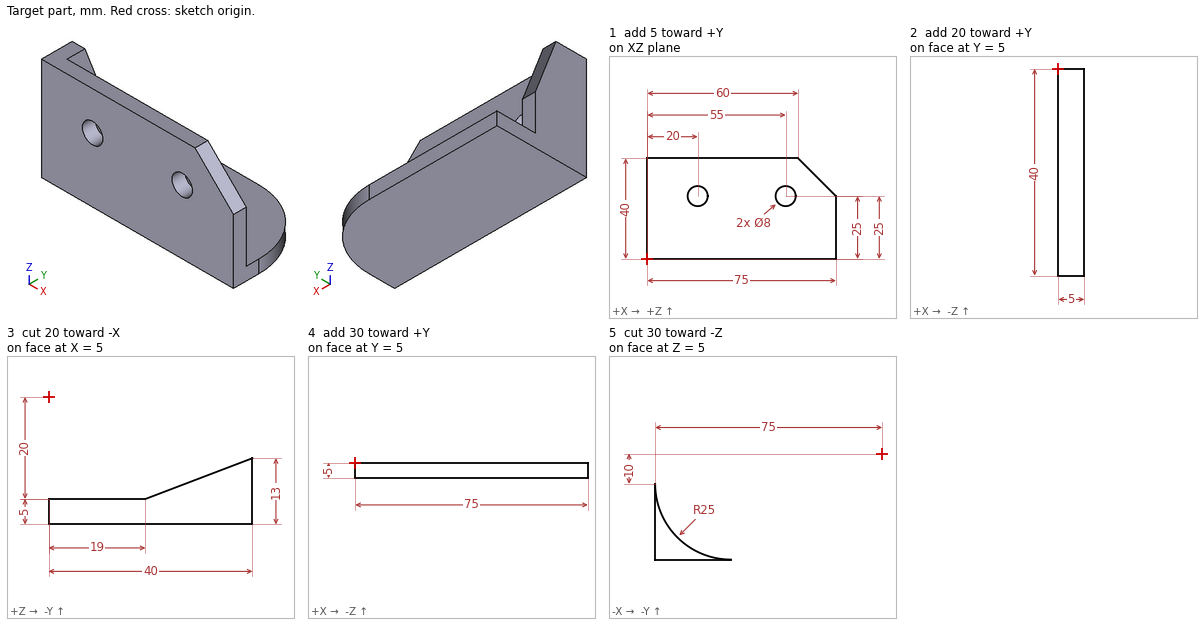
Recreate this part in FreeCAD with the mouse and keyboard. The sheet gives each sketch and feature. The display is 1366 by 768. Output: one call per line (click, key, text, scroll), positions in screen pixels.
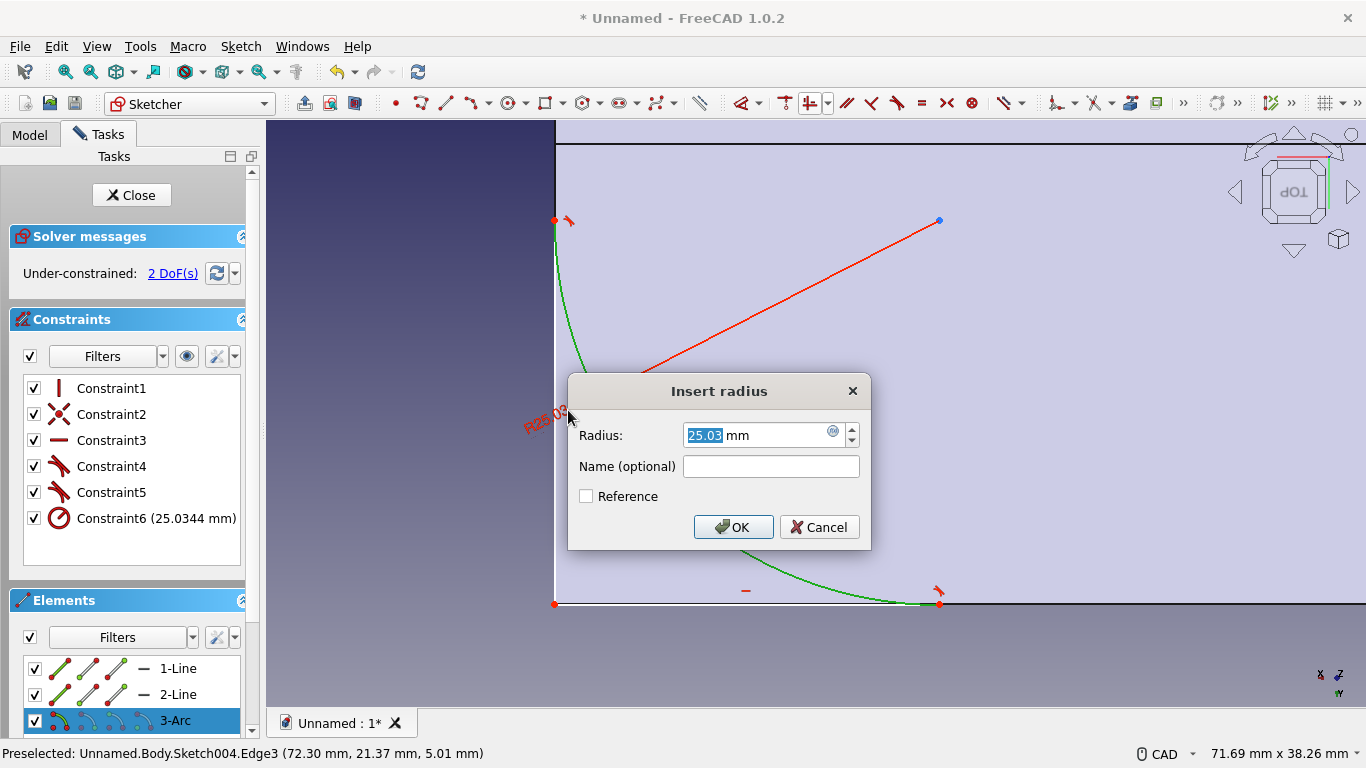
text(25)
key(Return)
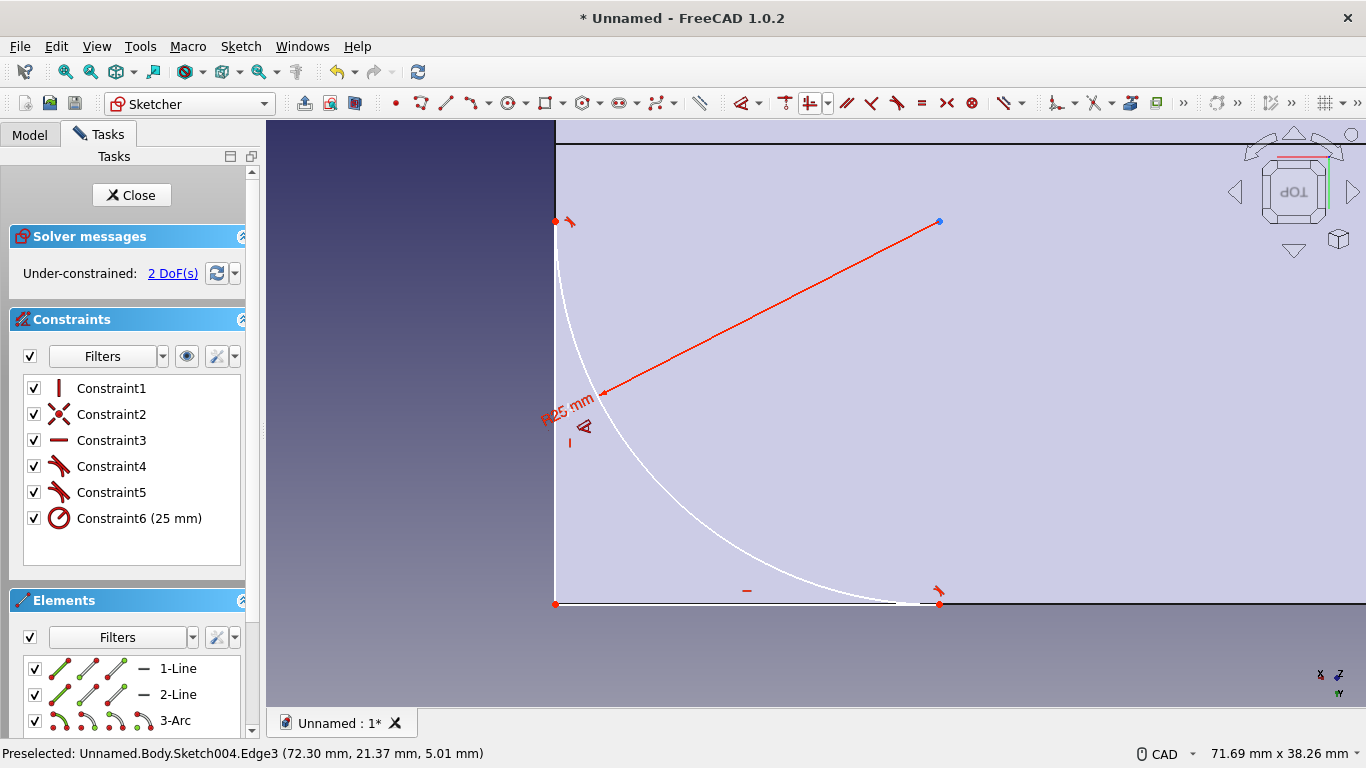
click(555, 221)
click(878, 255)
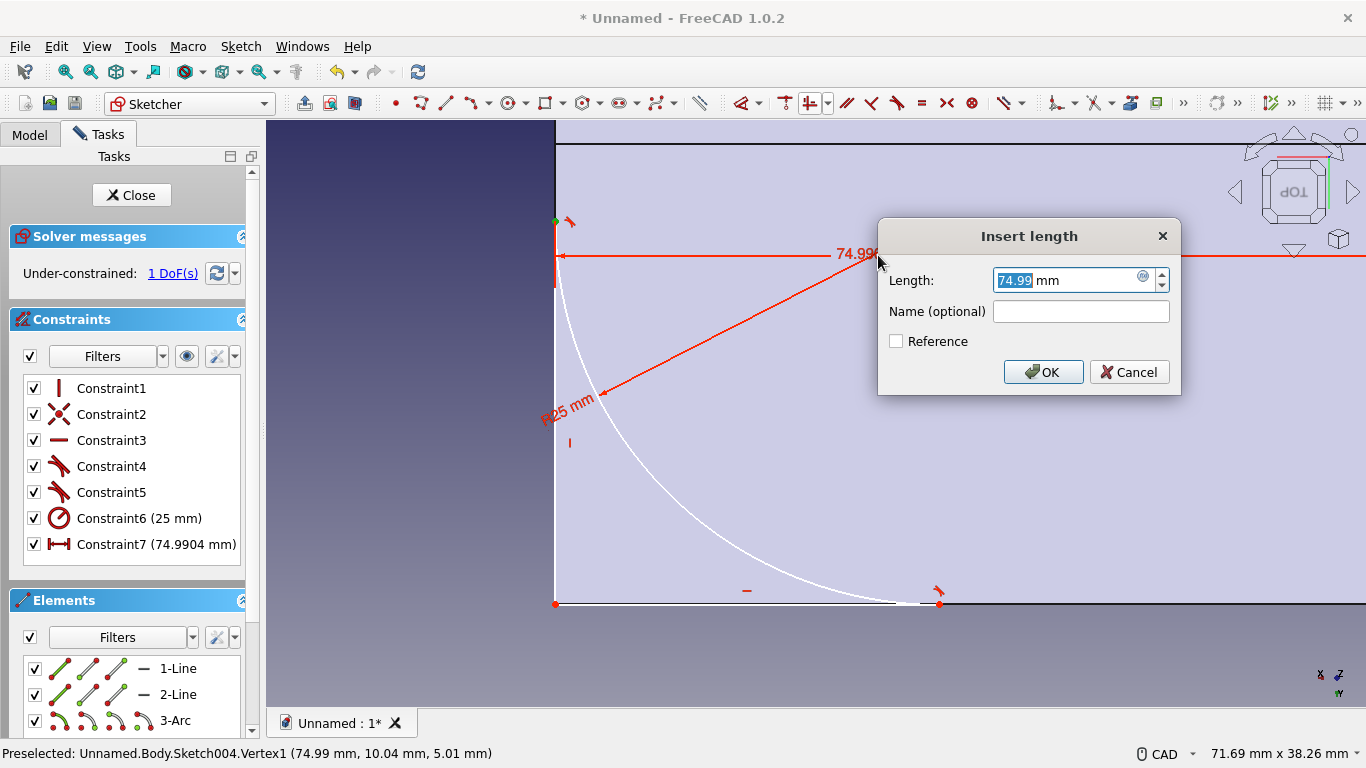
text(75)
key(Return)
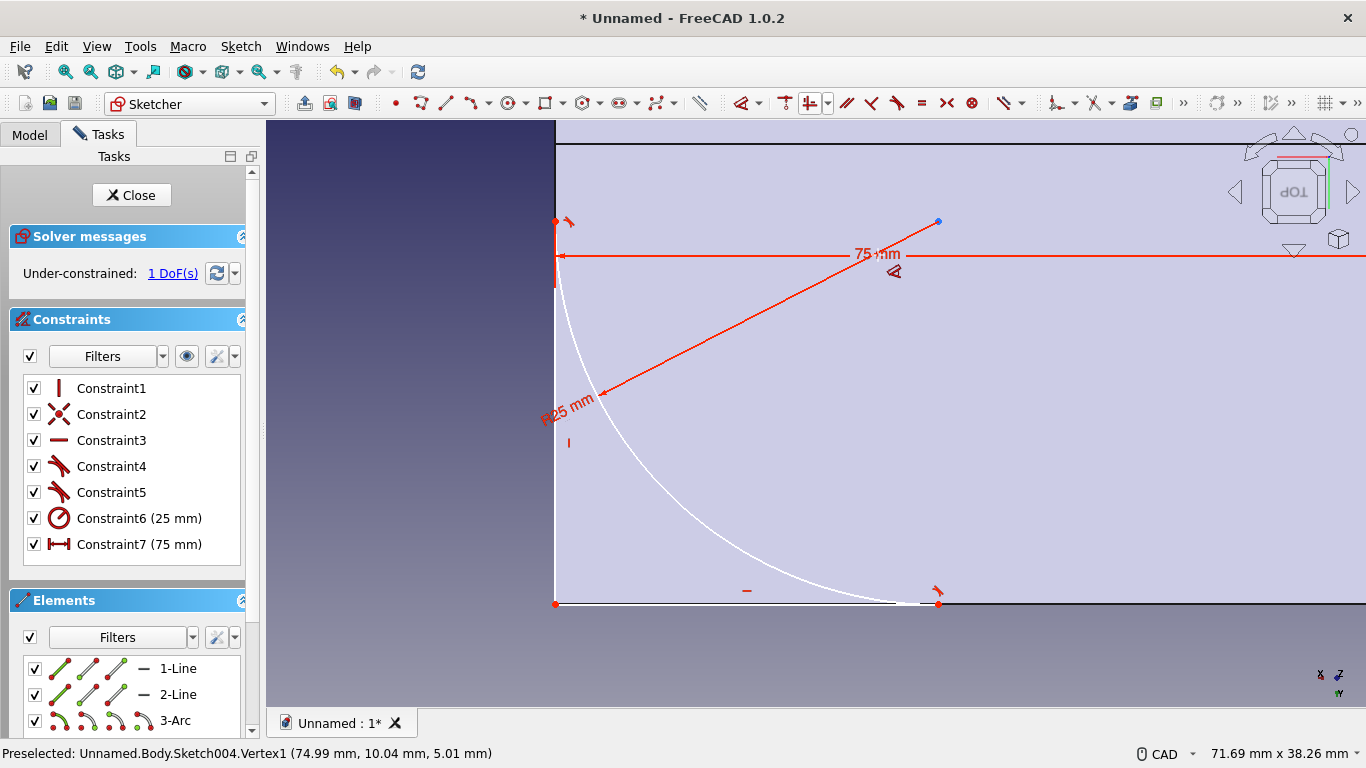
click(555, 221)
click(521, 185)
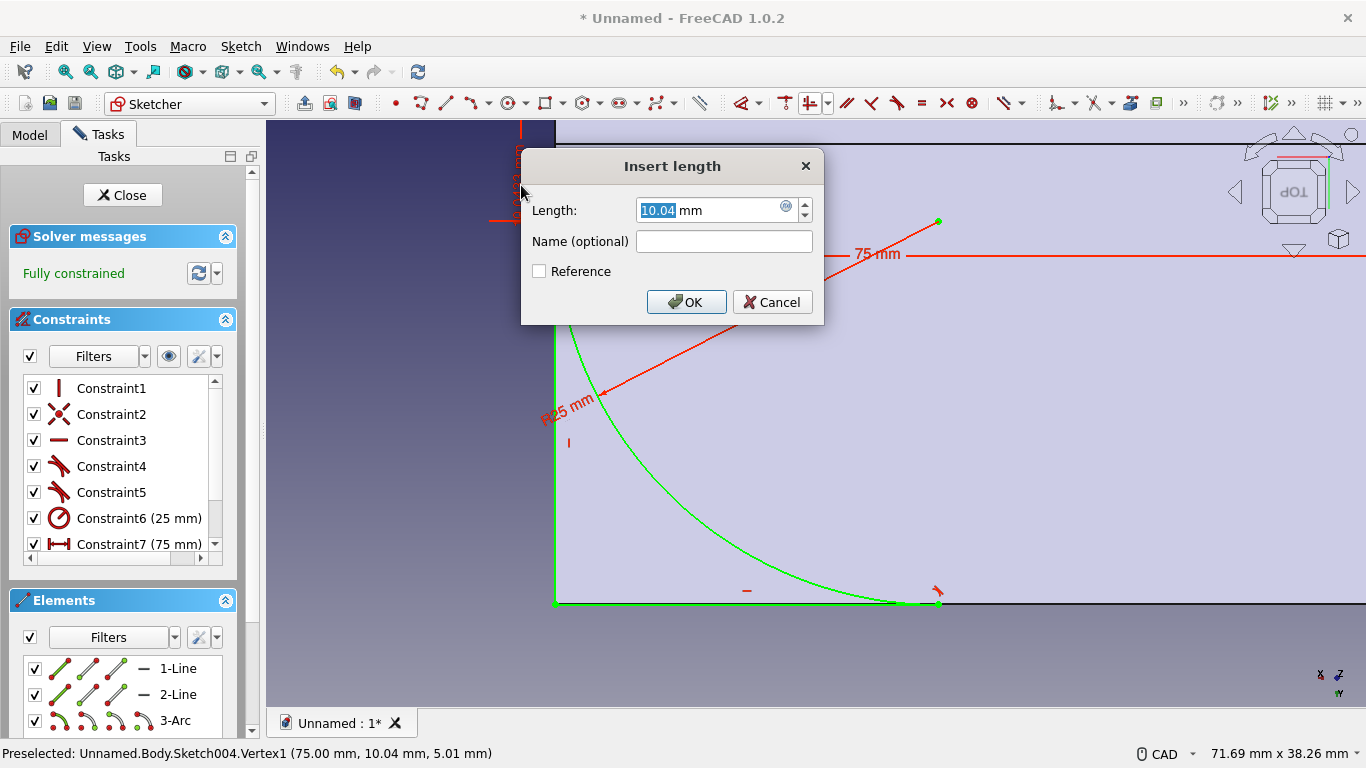
text(10)
key(Return)
key(Escape)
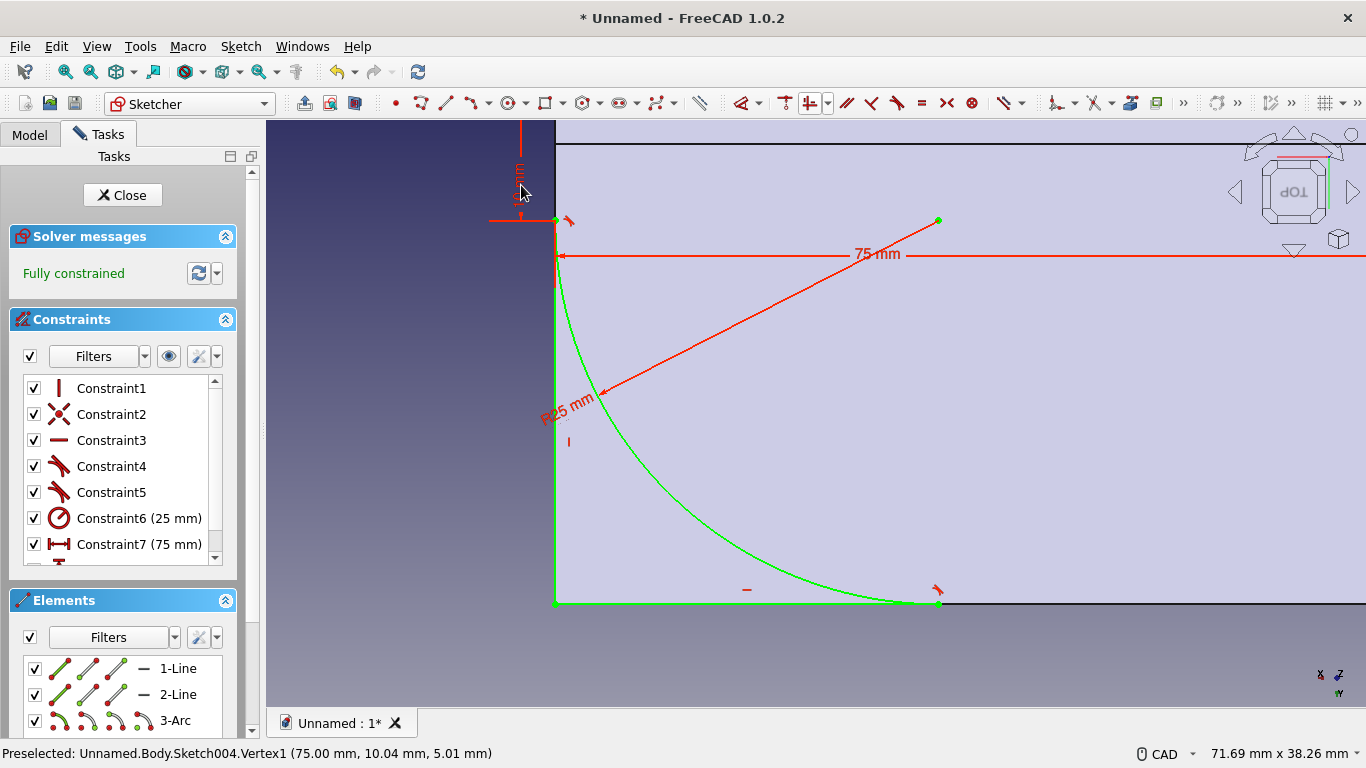
click(123, 195)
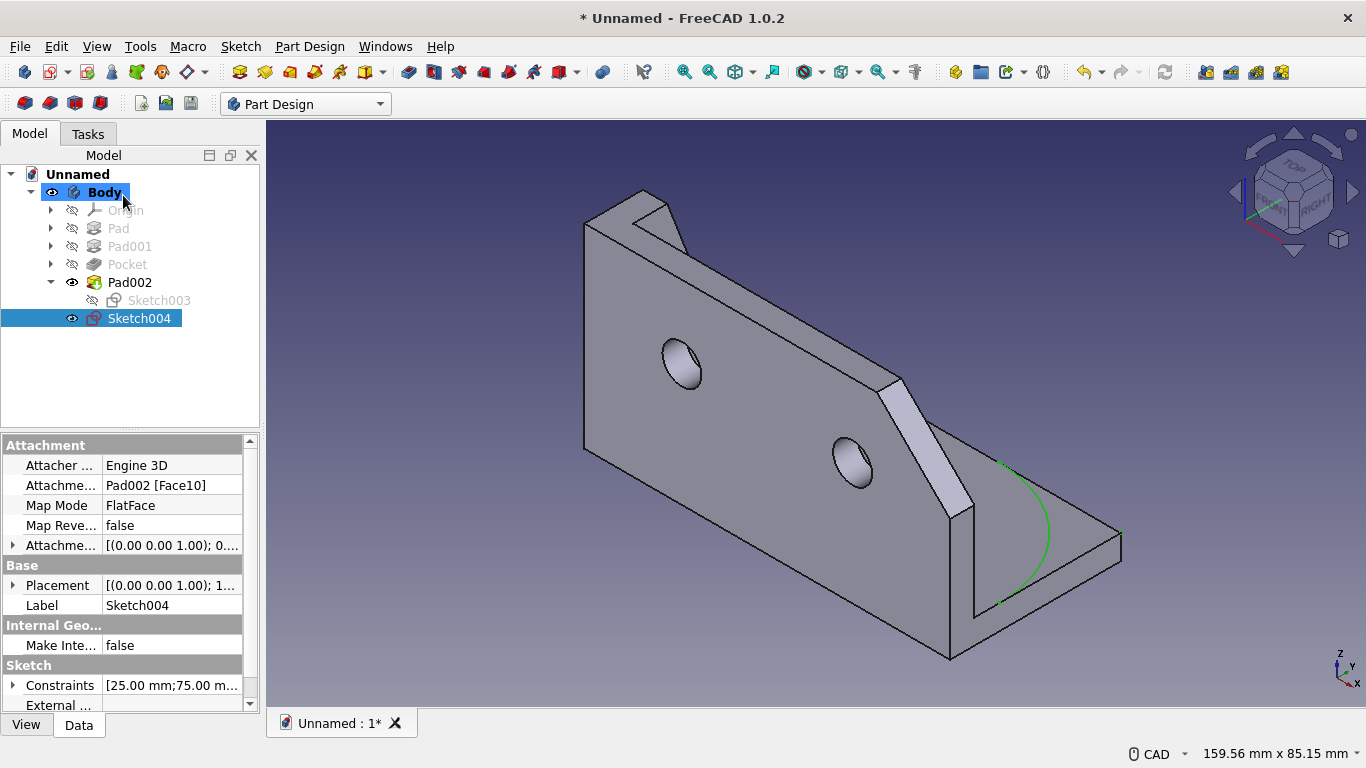
click(409, 72)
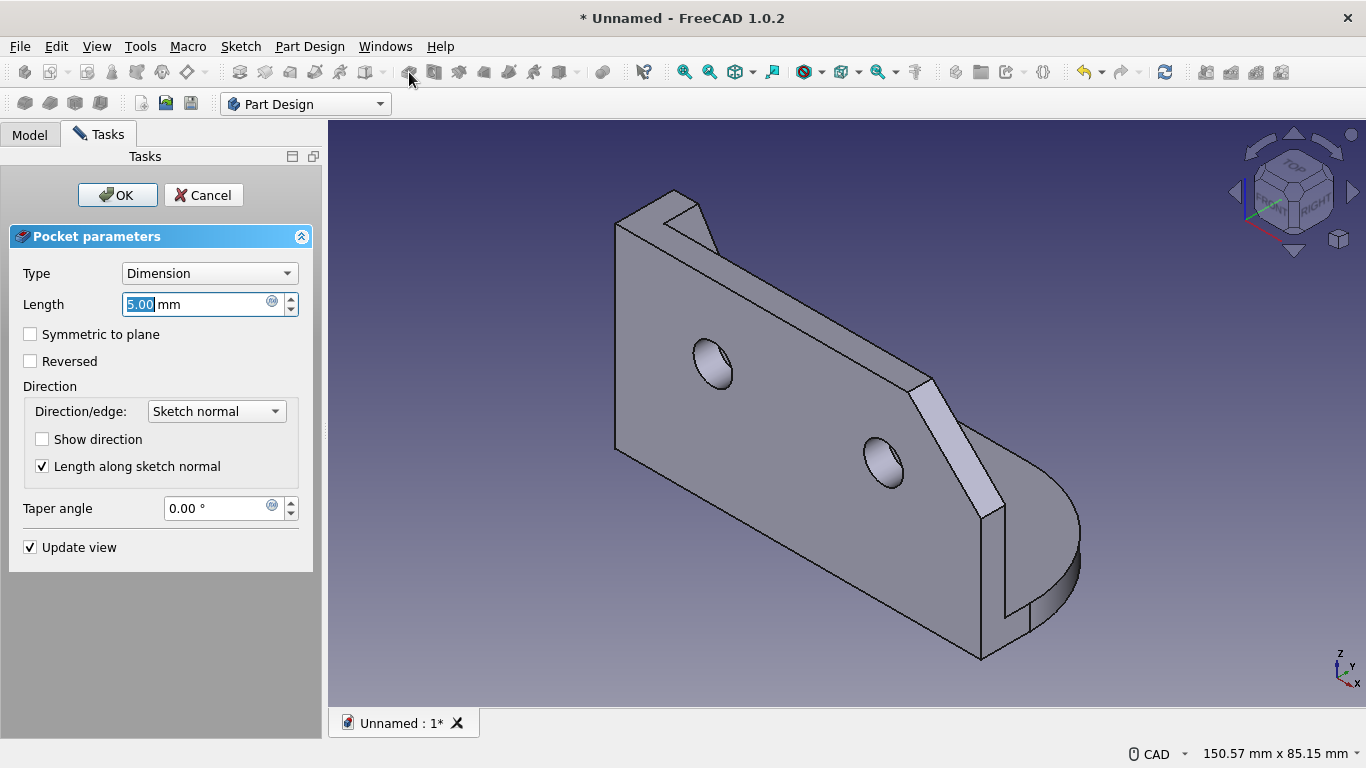
text(30)
key(Tab)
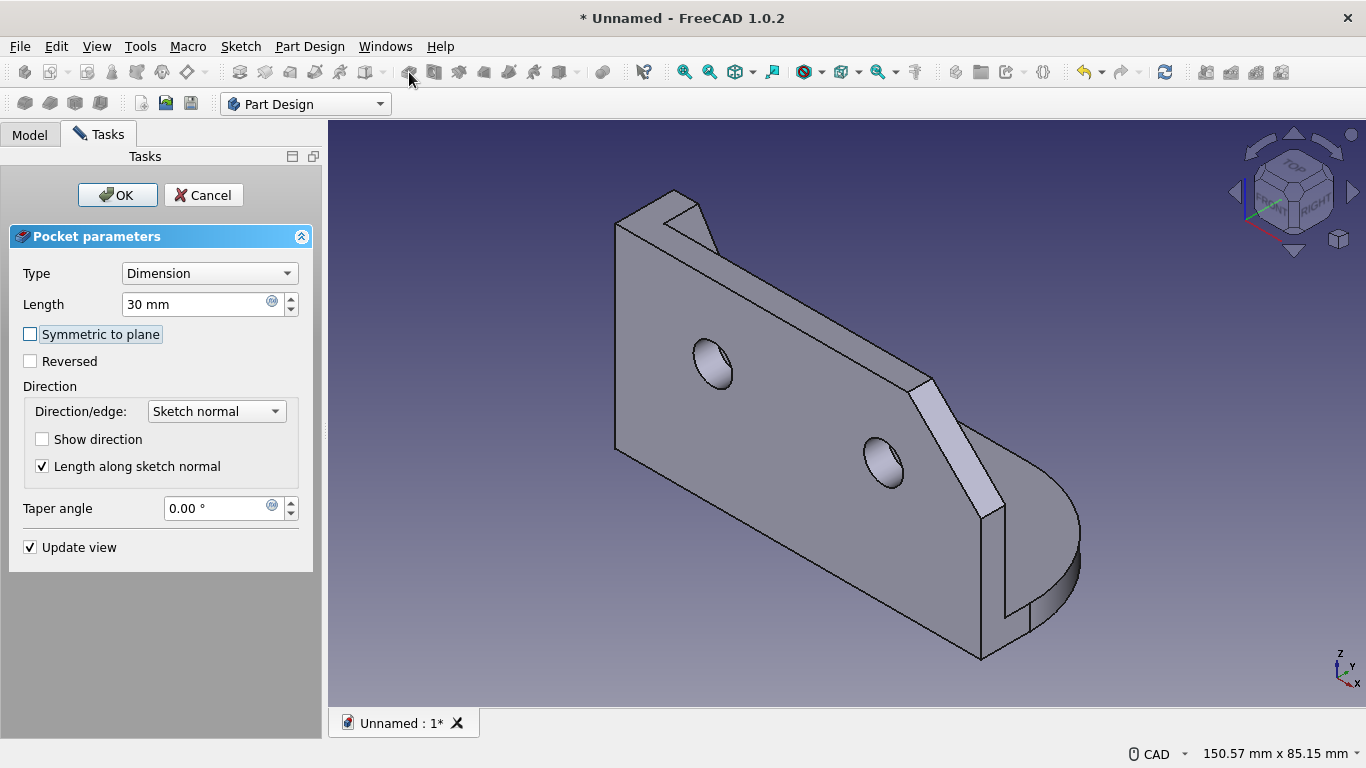
click(118, 195)